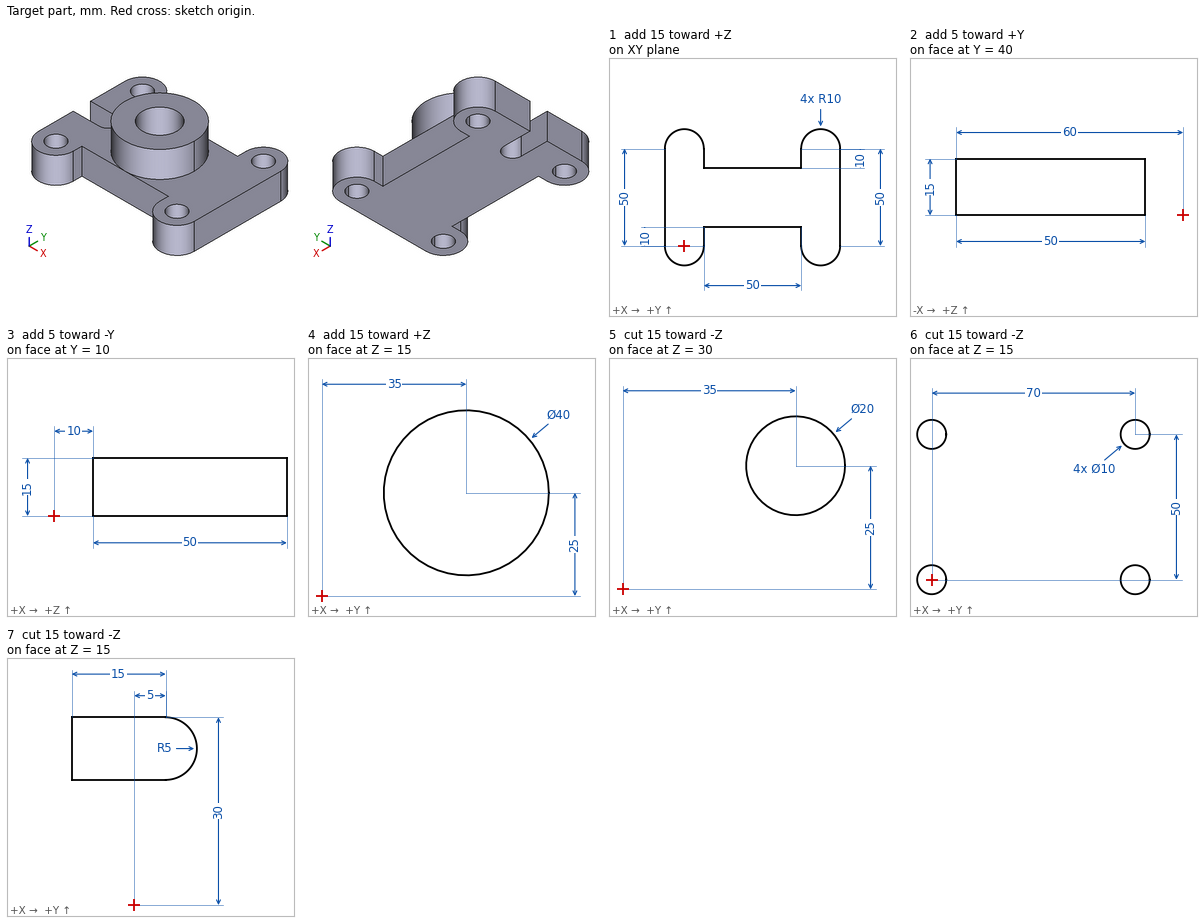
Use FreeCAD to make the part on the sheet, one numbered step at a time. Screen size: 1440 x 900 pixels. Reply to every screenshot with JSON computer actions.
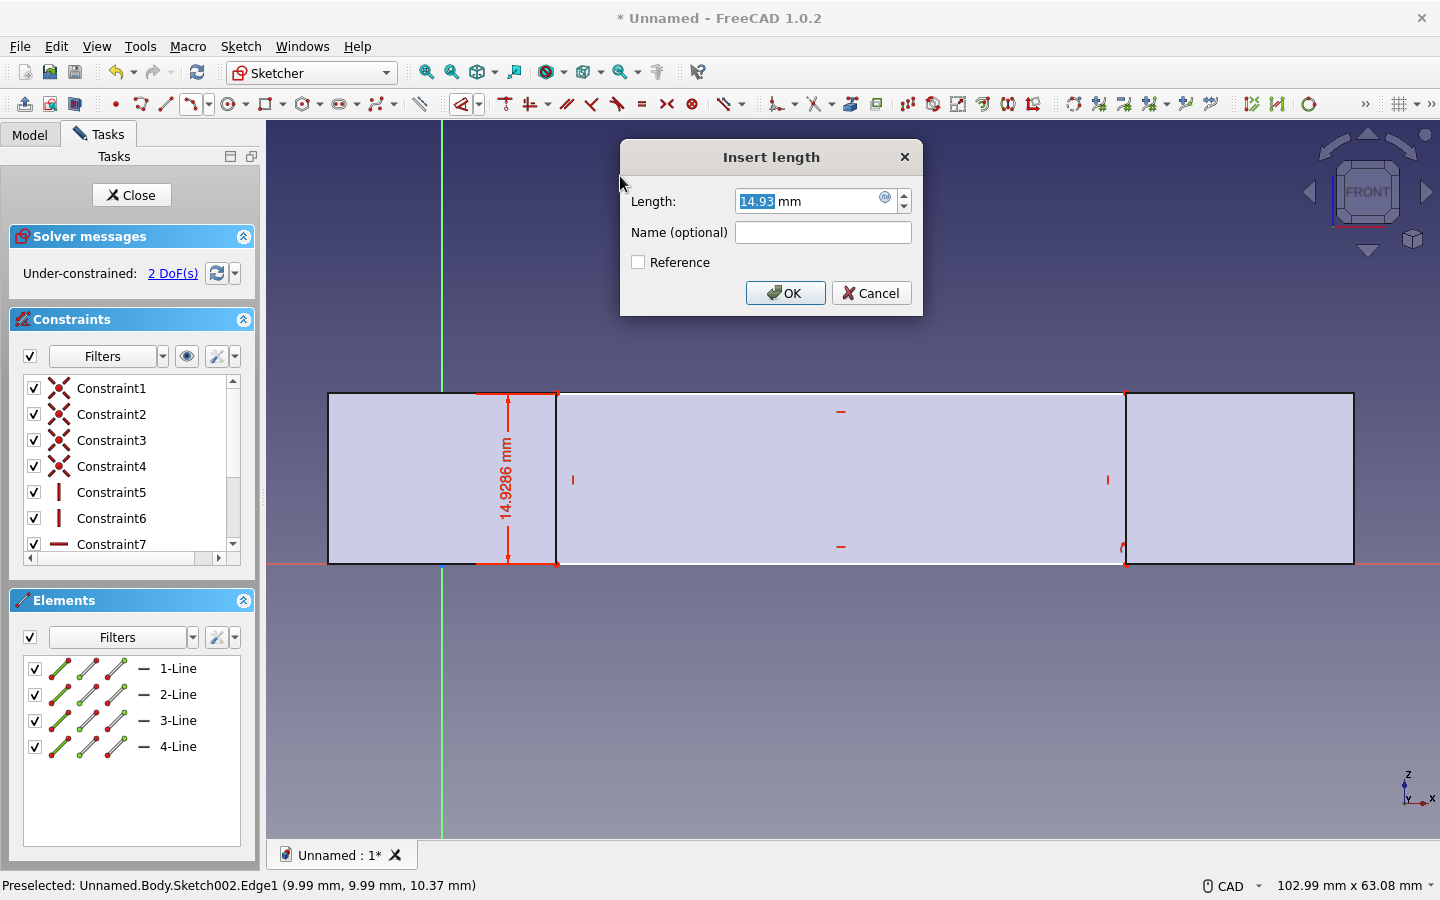
{"action": "type", "text": "15"}
{"action": "key", "text": "Return"}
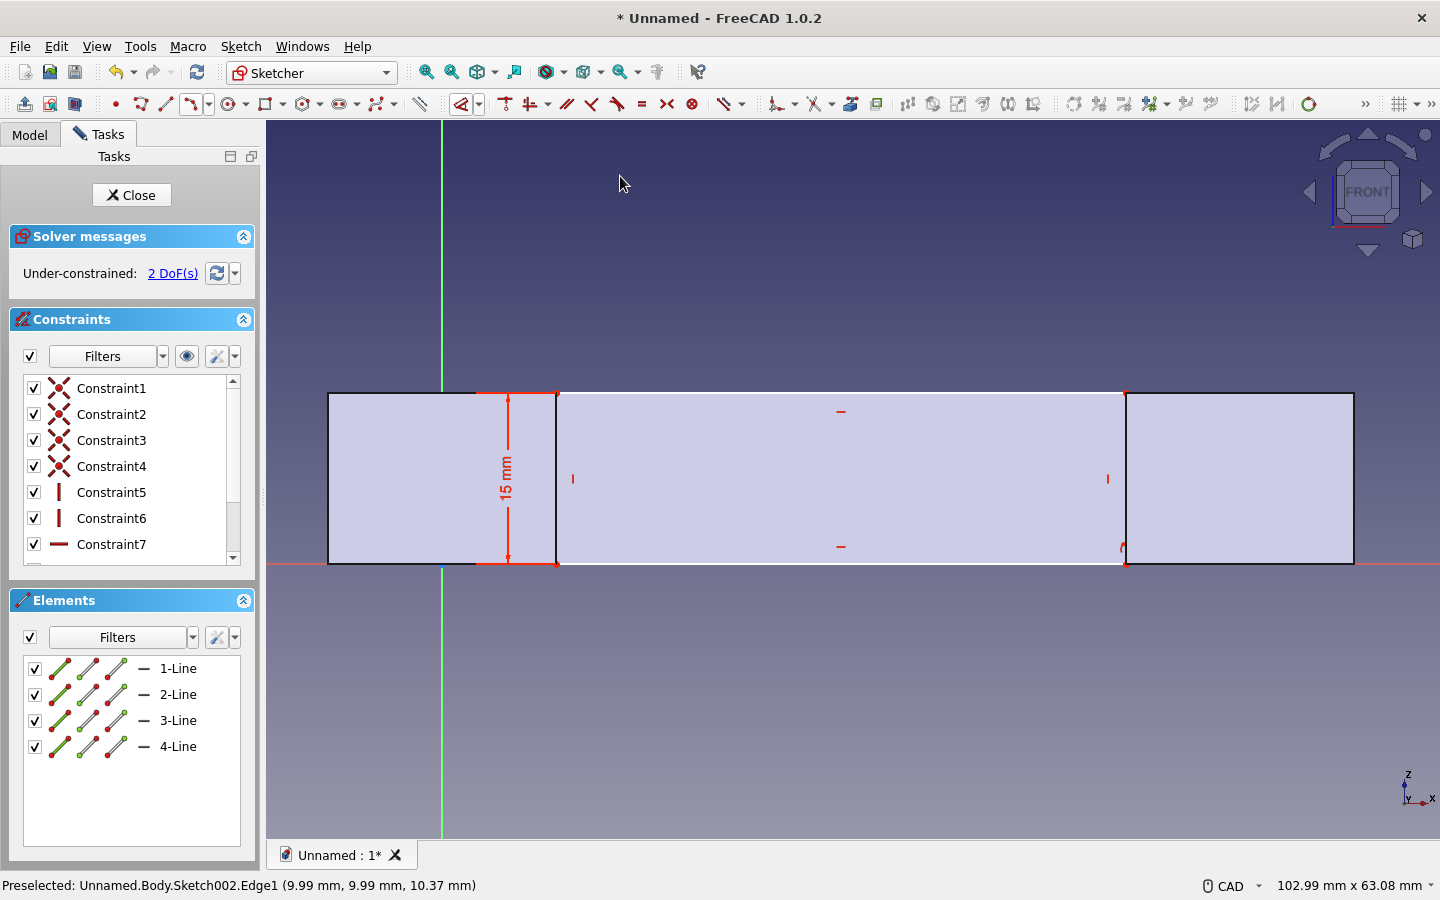
{"action": "left_click", "coordinate": [727, 564]}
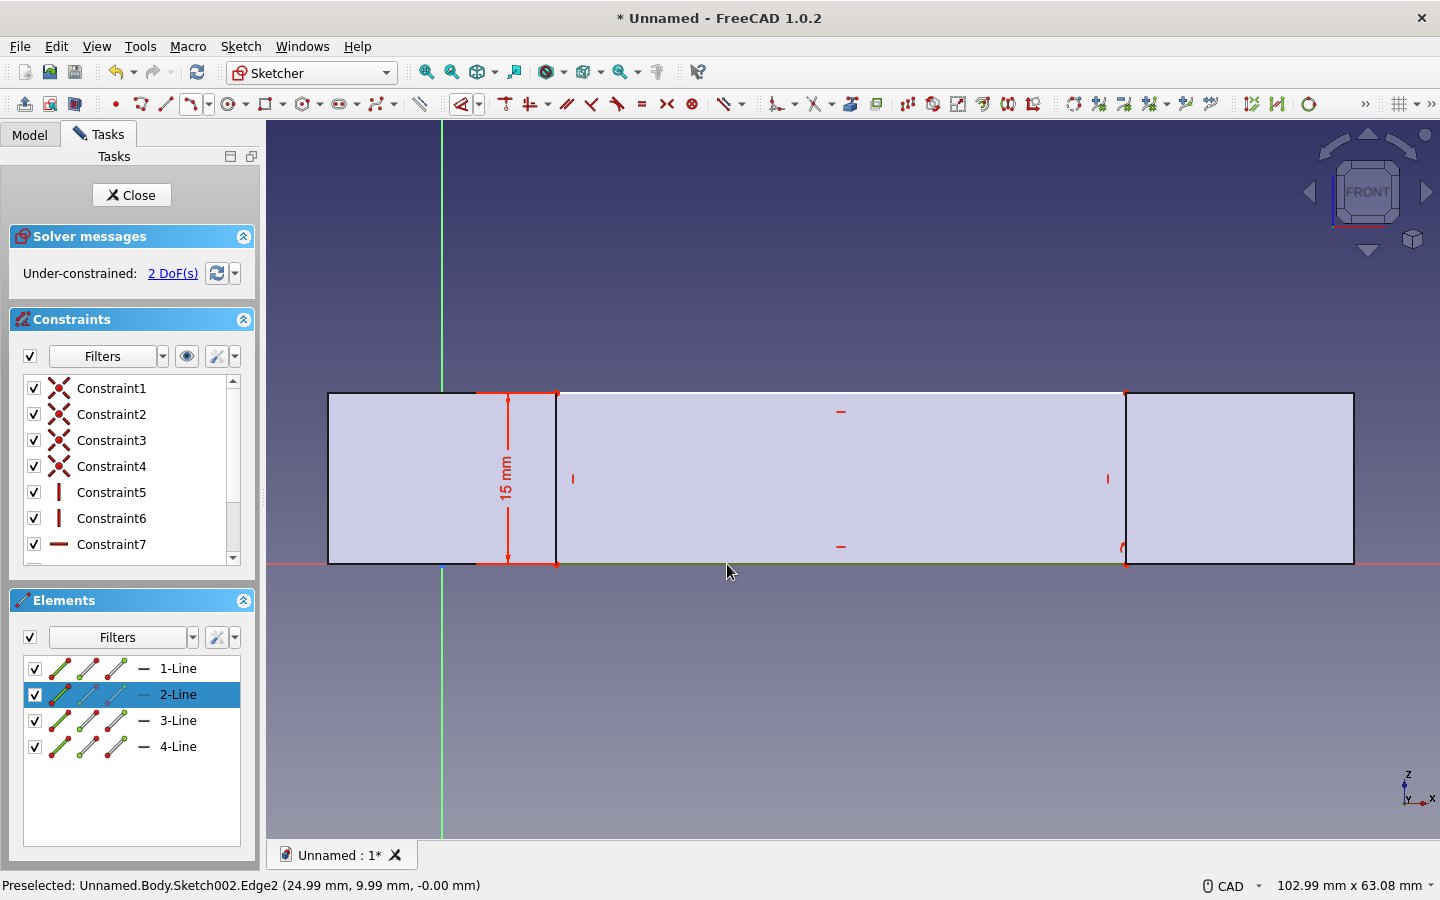
{"action": "left_click", "coordinate": [478, 104]}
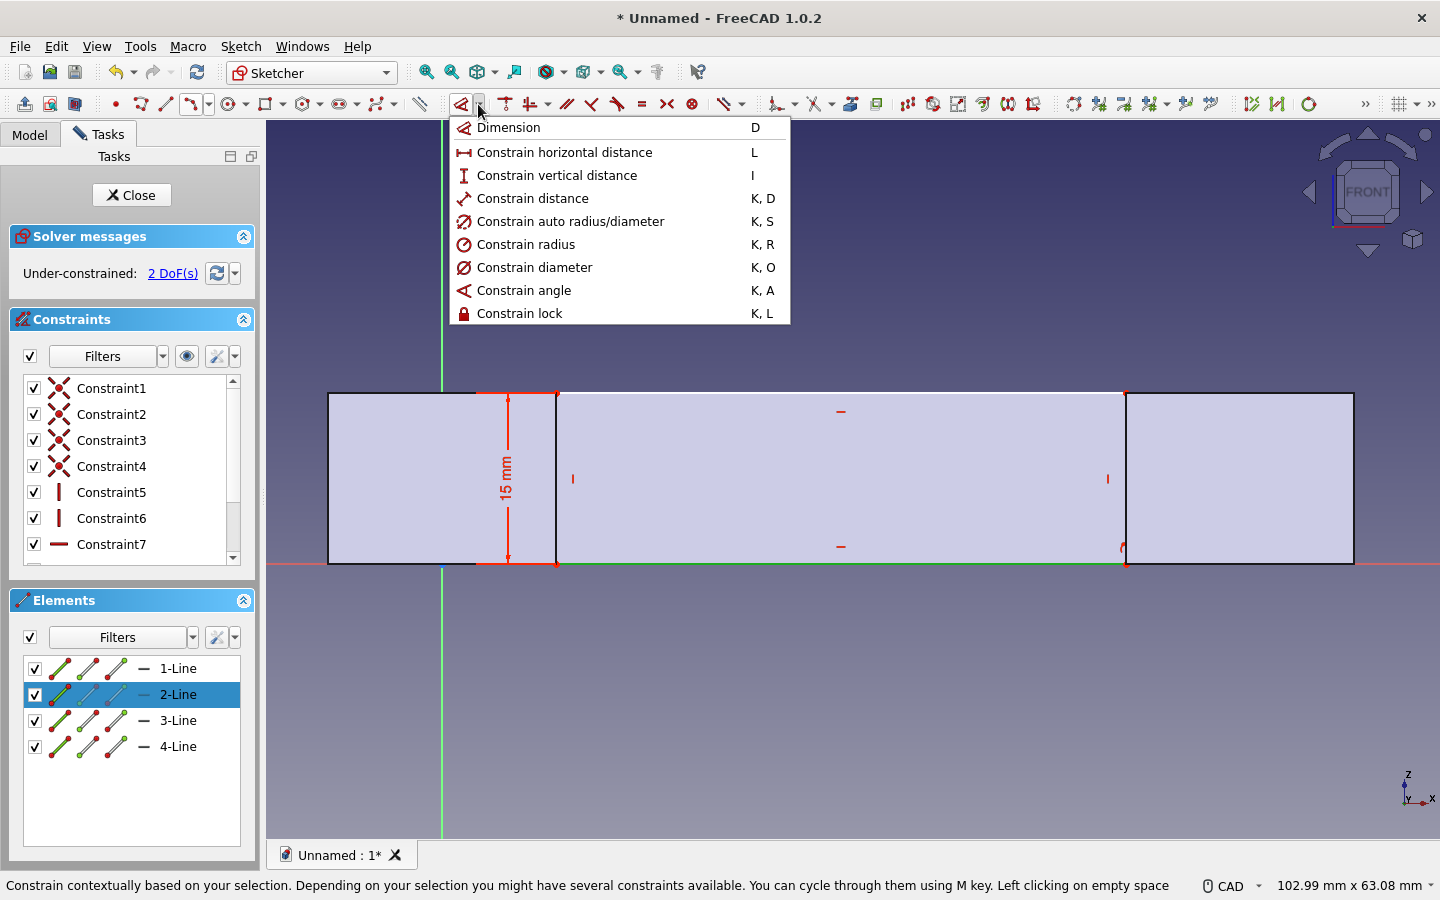
{"action": "left_click", "coordinate": [620, 152]}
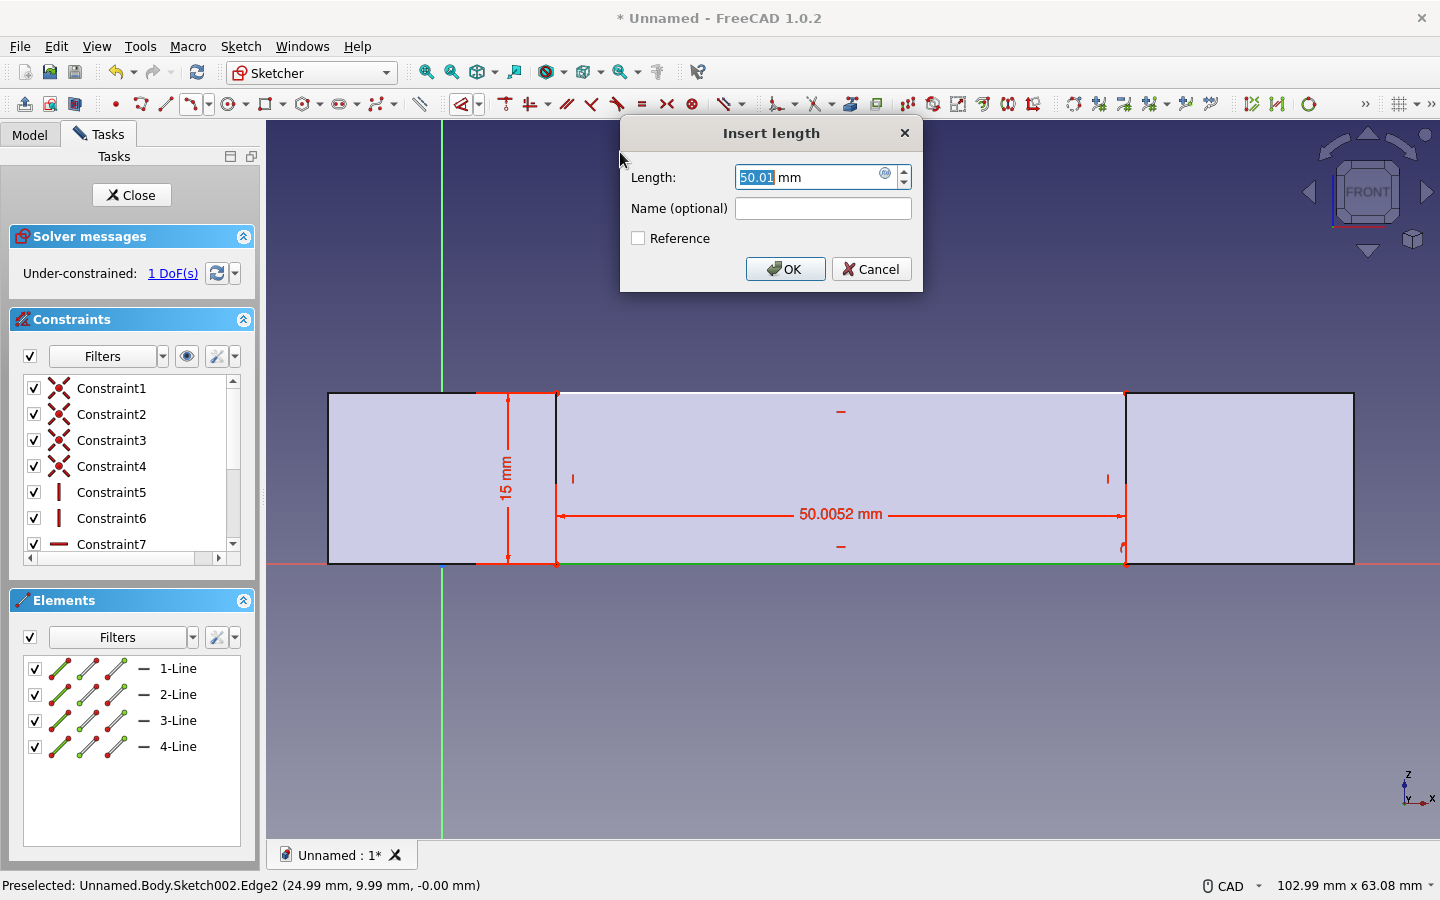
{"action": "type", "text": "50"}
{"action": "key", "text": "Return"}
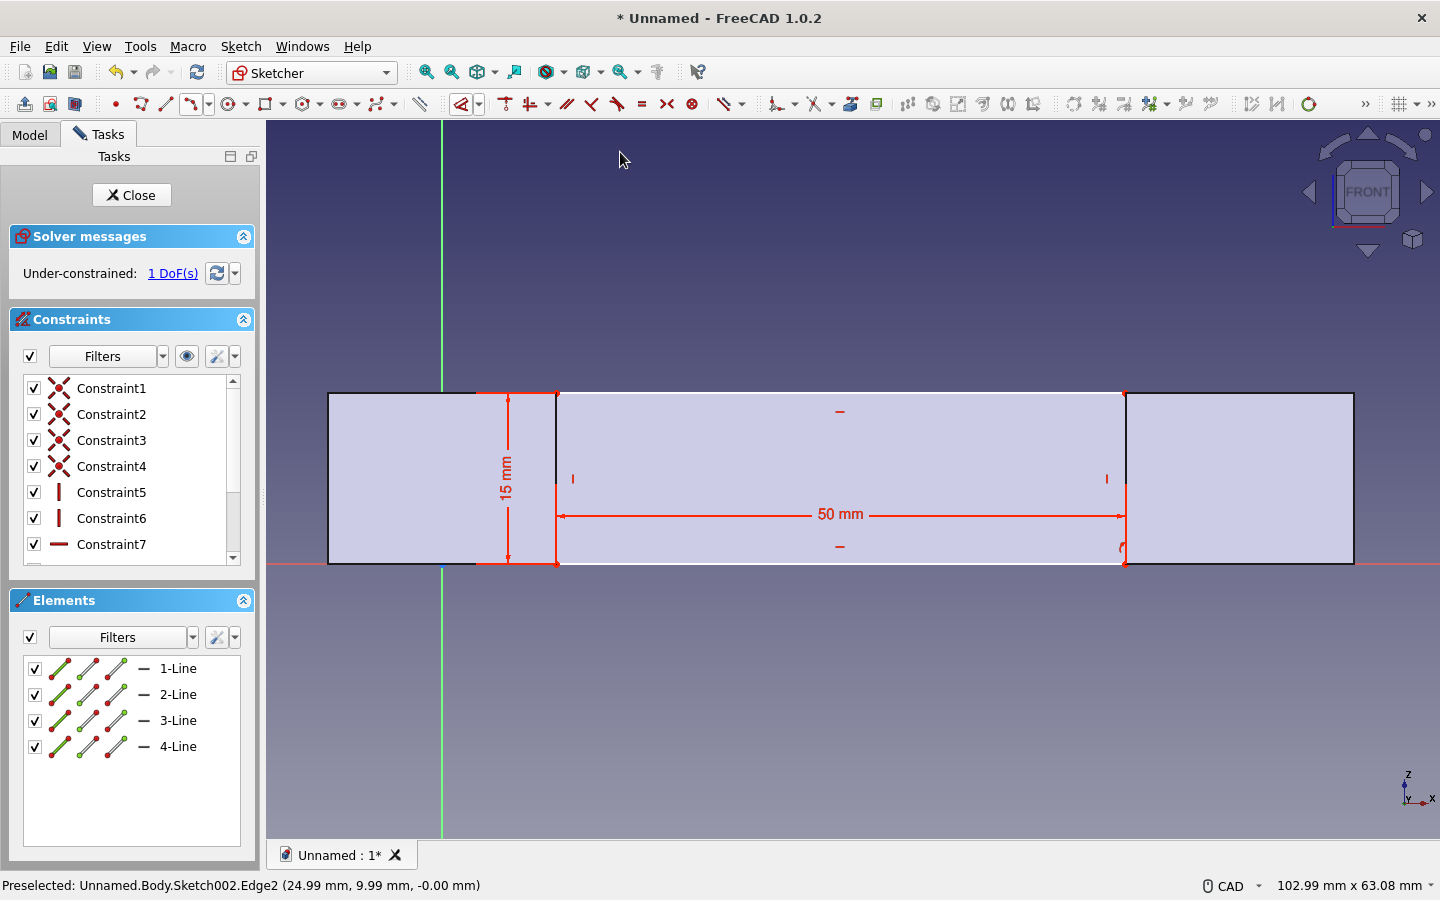
{"action": "left_click", "coordinate": [556, 393]}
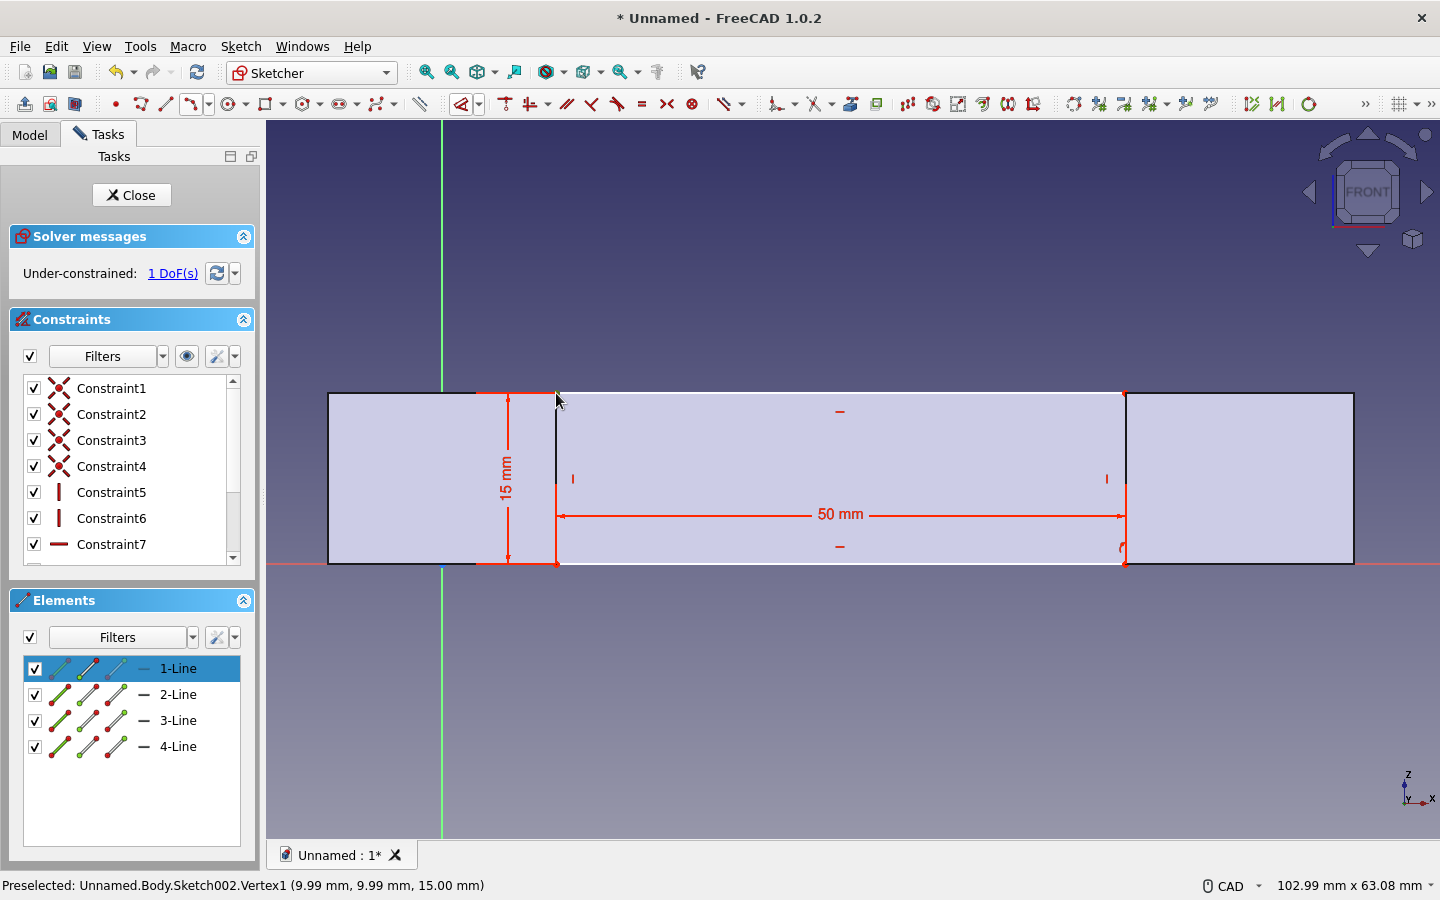
{"action": "left_click", "coordinate": [478, 104]}